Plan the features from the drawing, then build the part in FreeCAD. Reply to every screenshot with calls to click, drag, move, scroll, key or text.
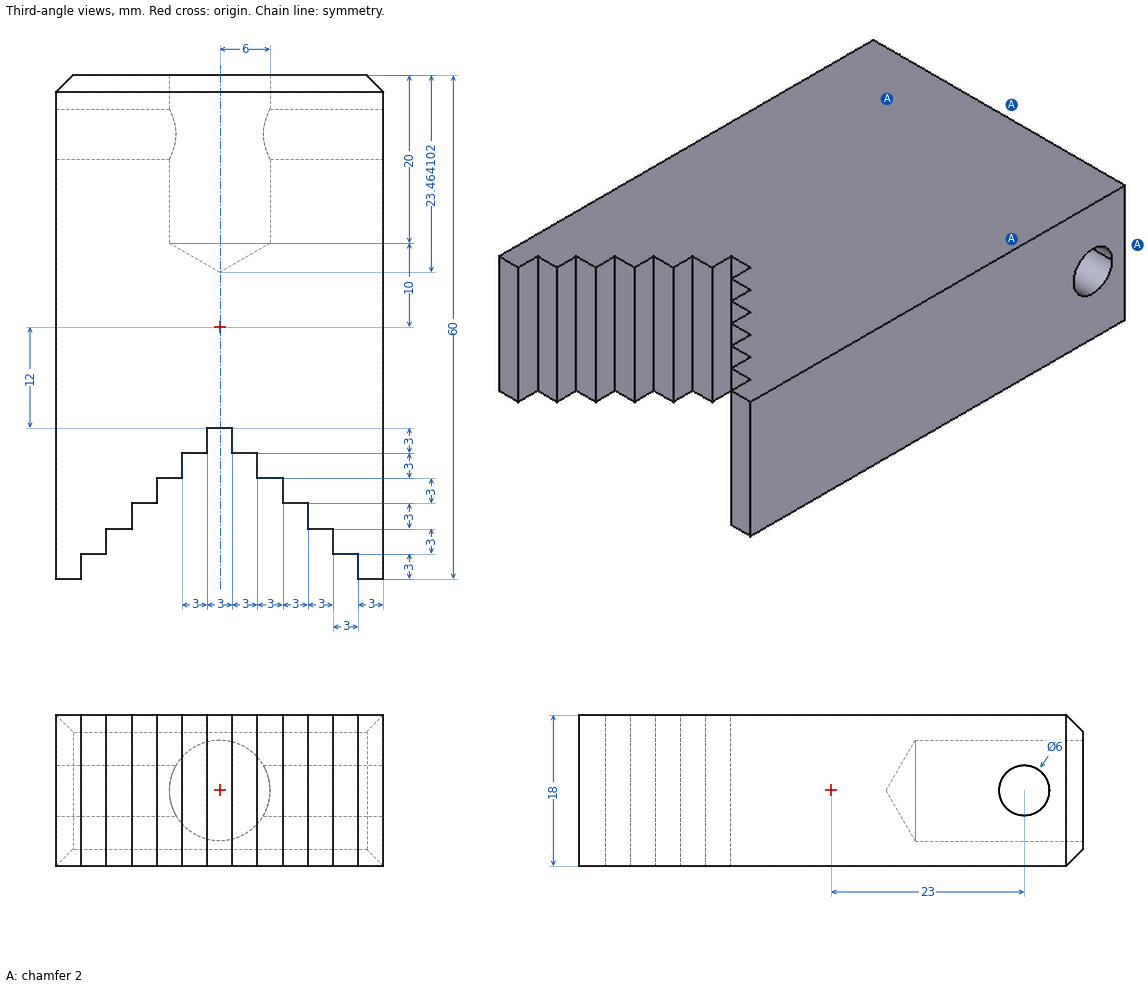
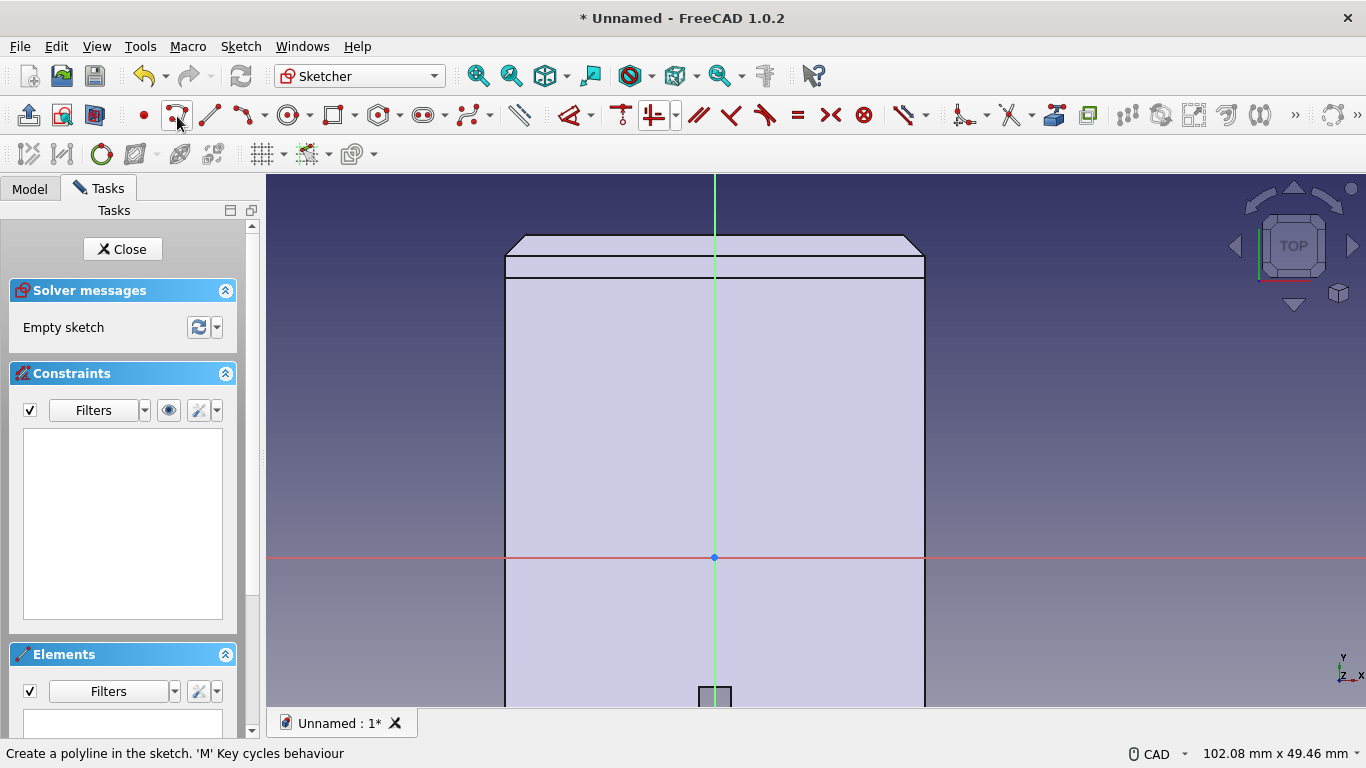
click(715, 487)
click(779, 450)
click(779, 235)
click(724, 235)
click(715, 488)
key(Escape)
key(Escape)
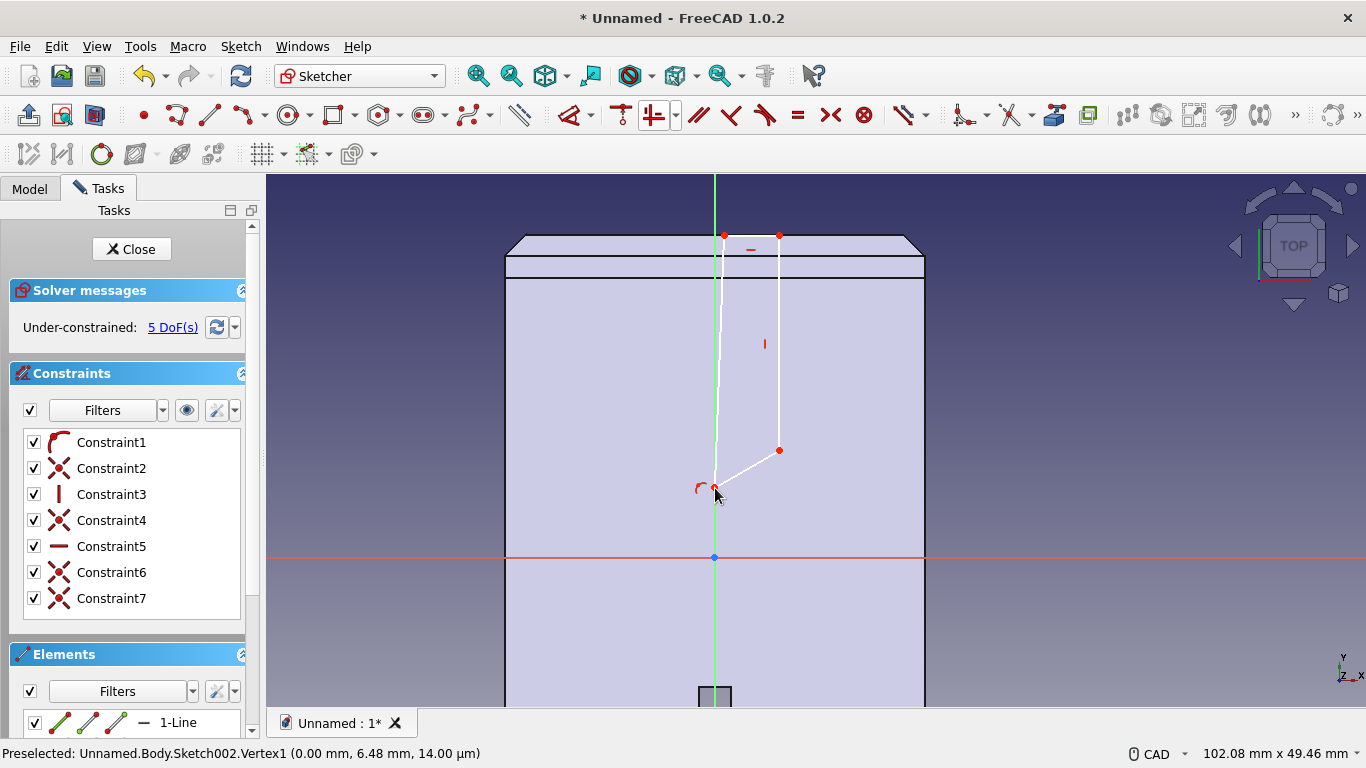
click(718, 412)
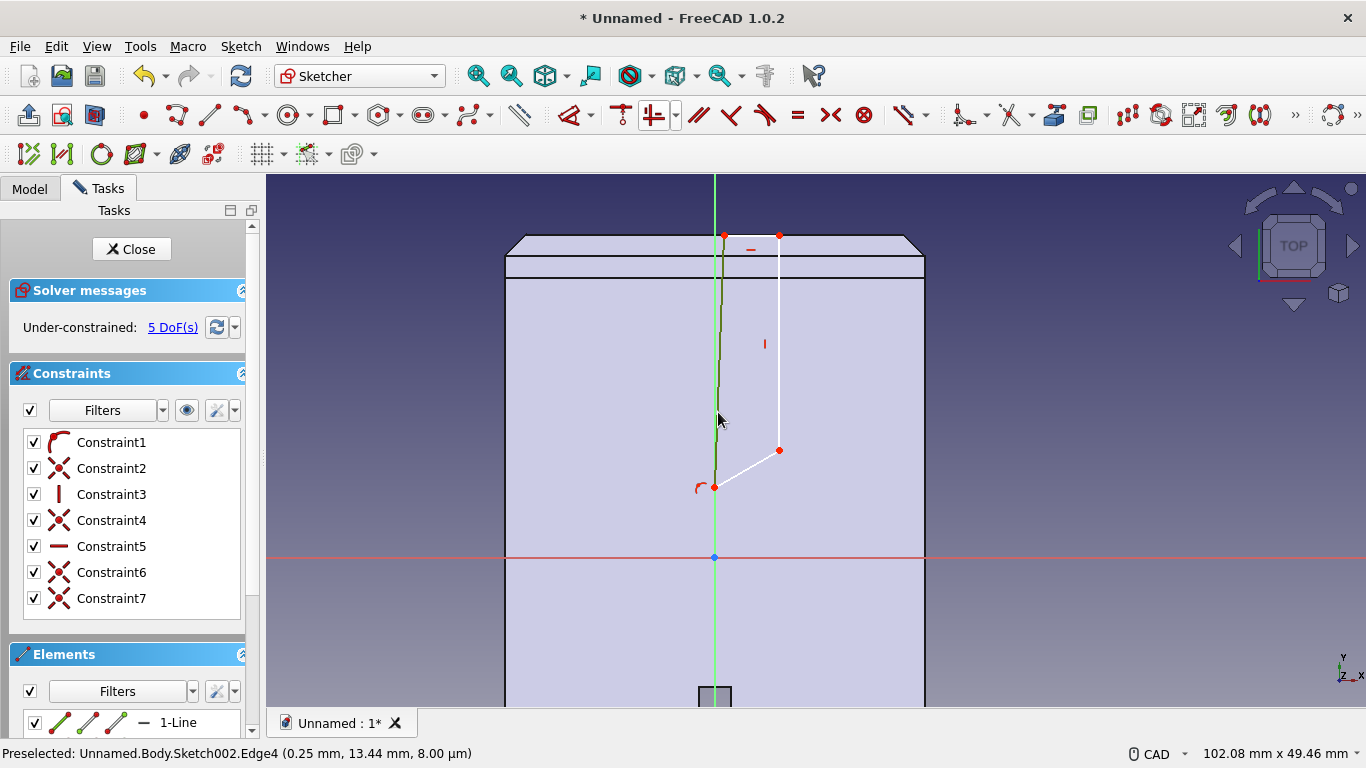
click(676, 116)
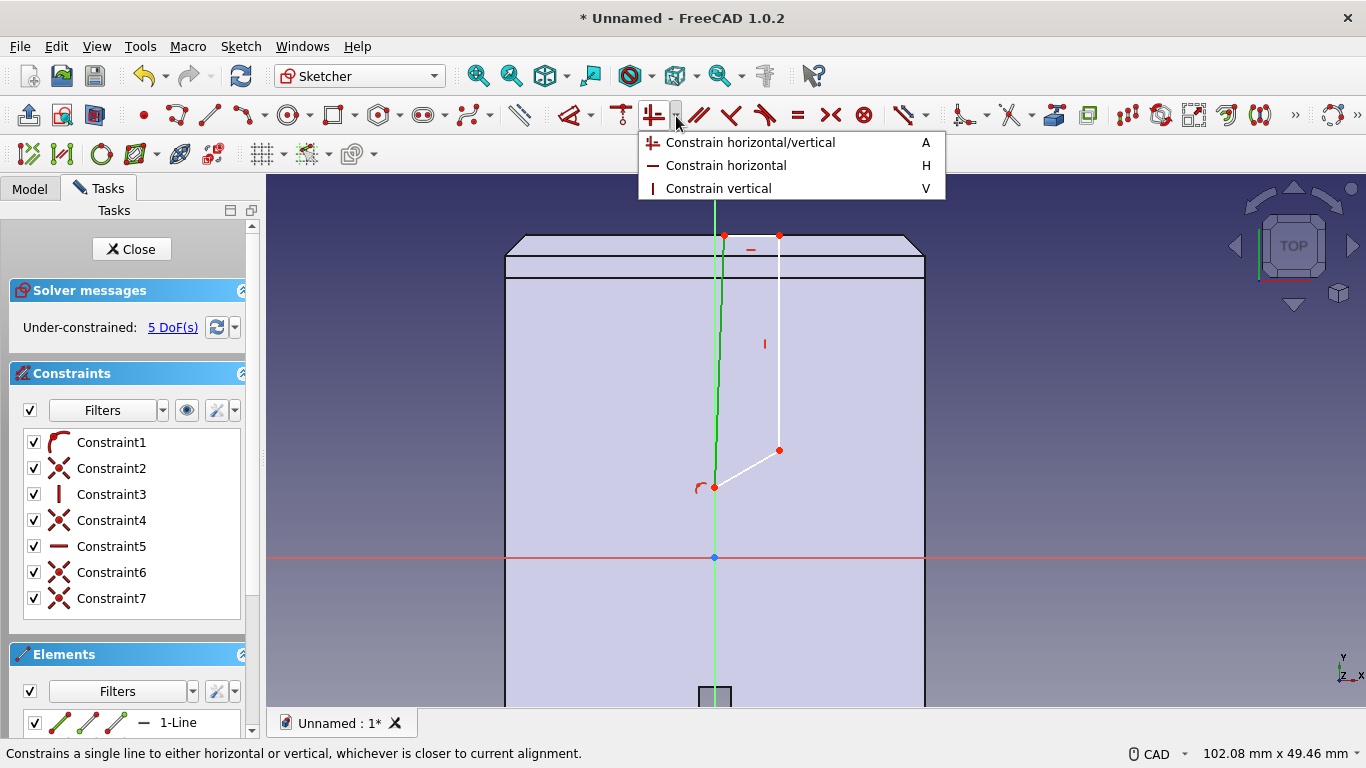
click(792, 188)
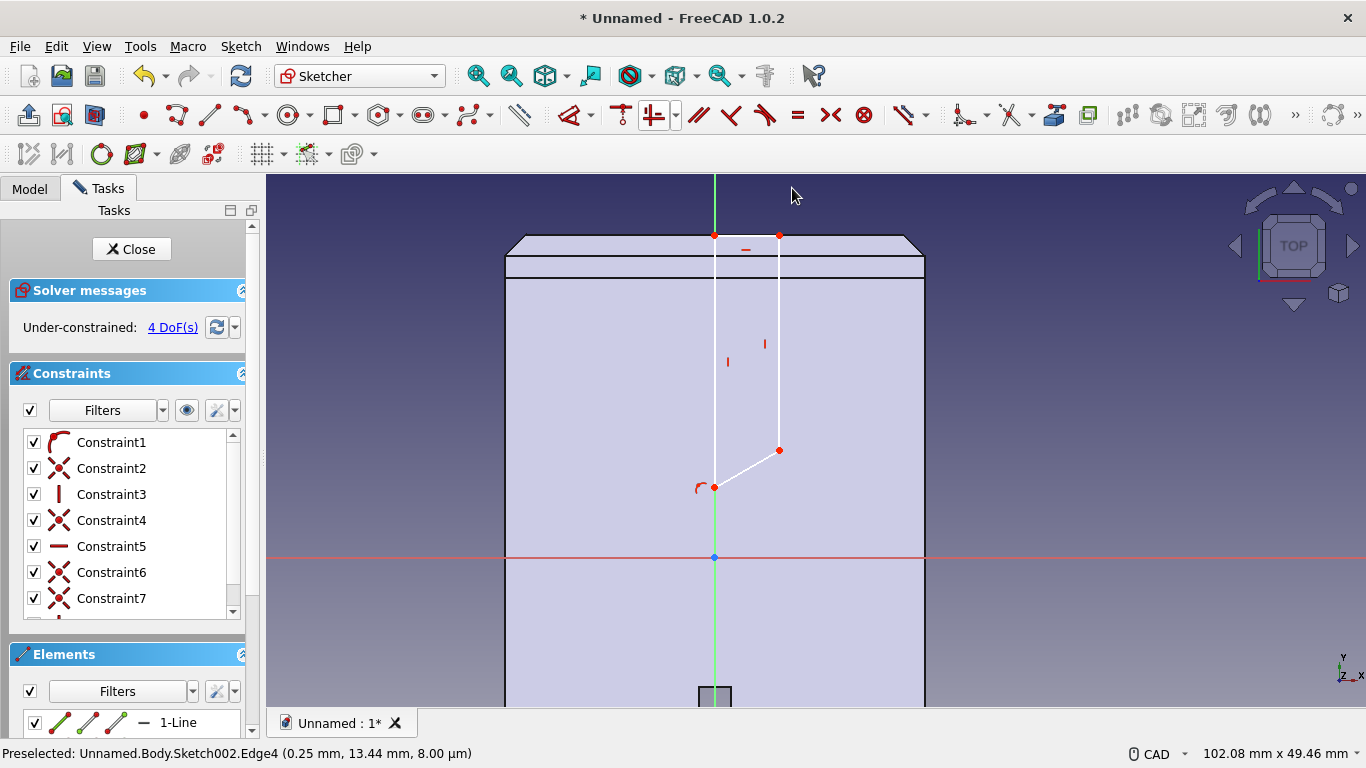
click(568, 116)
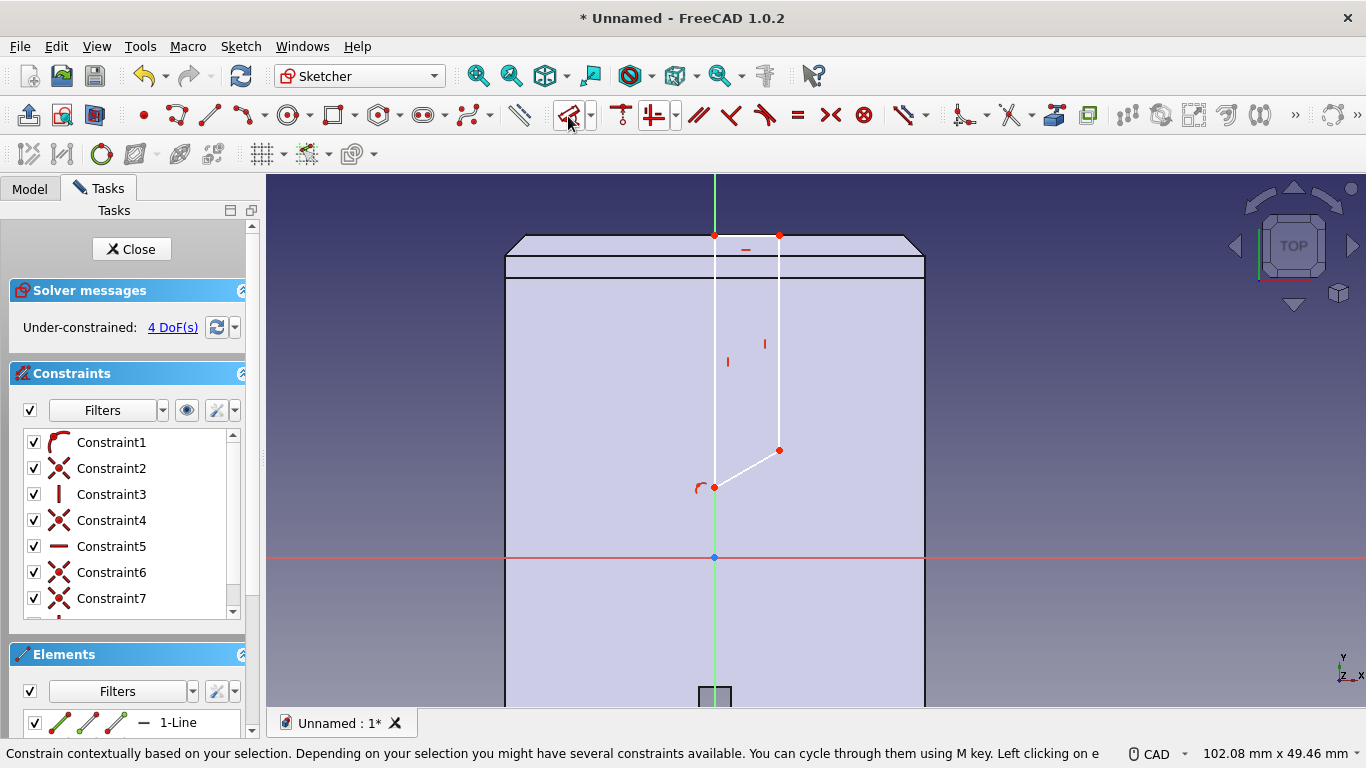
click(760, 236)
click(747, 270)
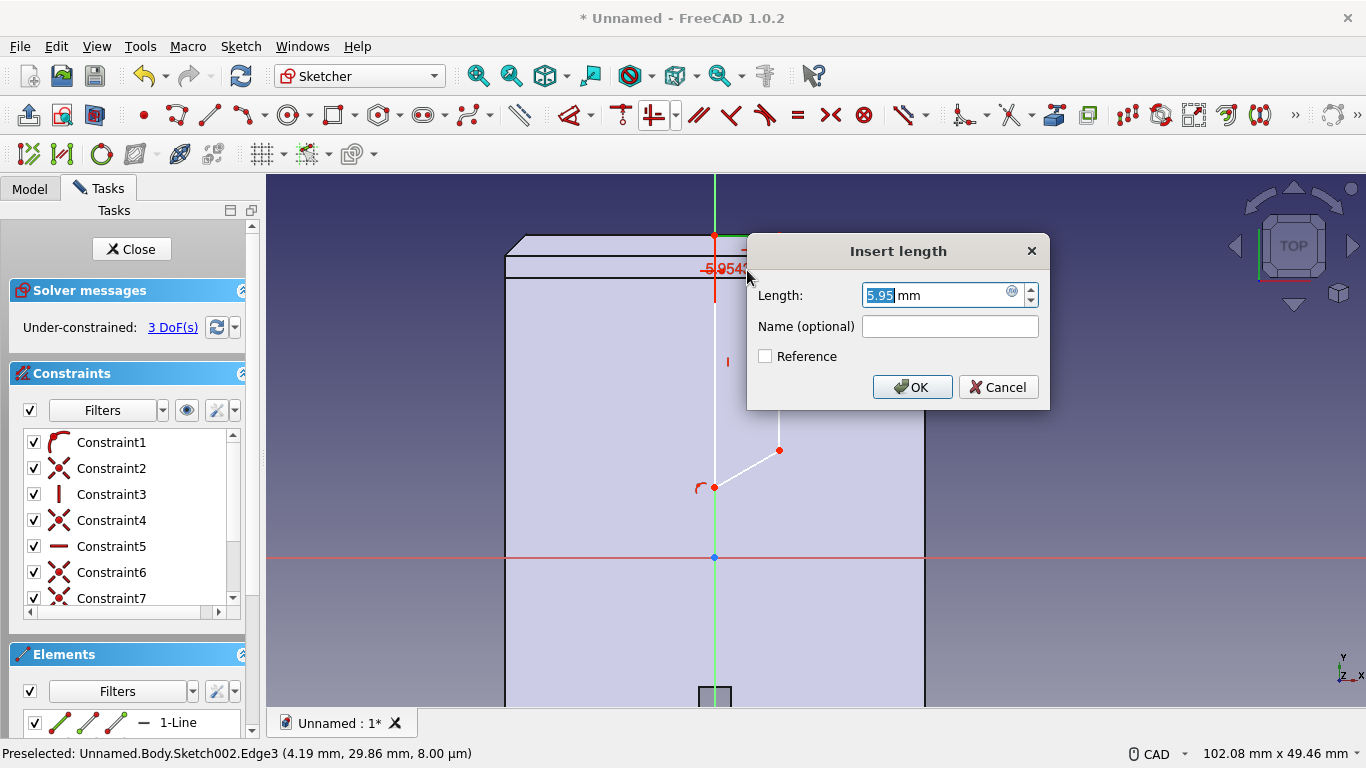
text(6)
key(Return)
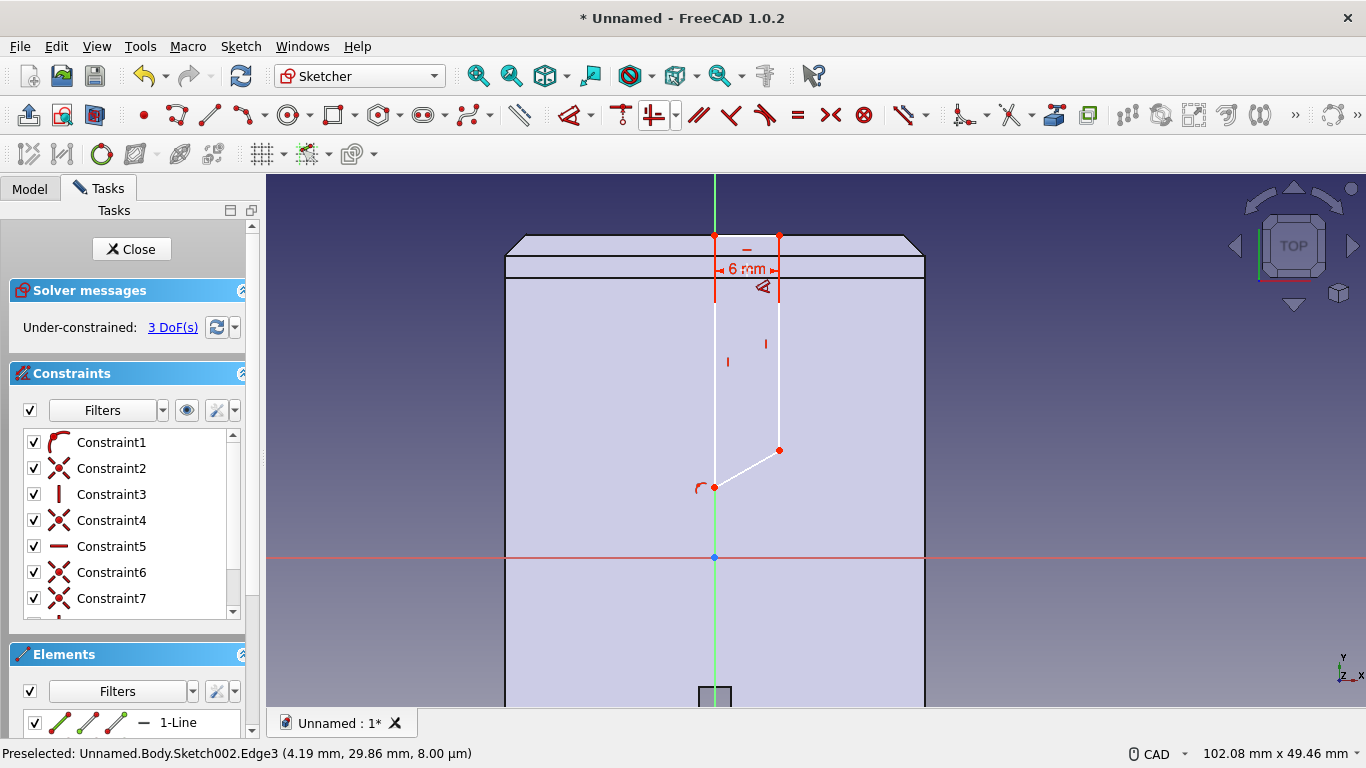
click(779, 386)
click(813, 343)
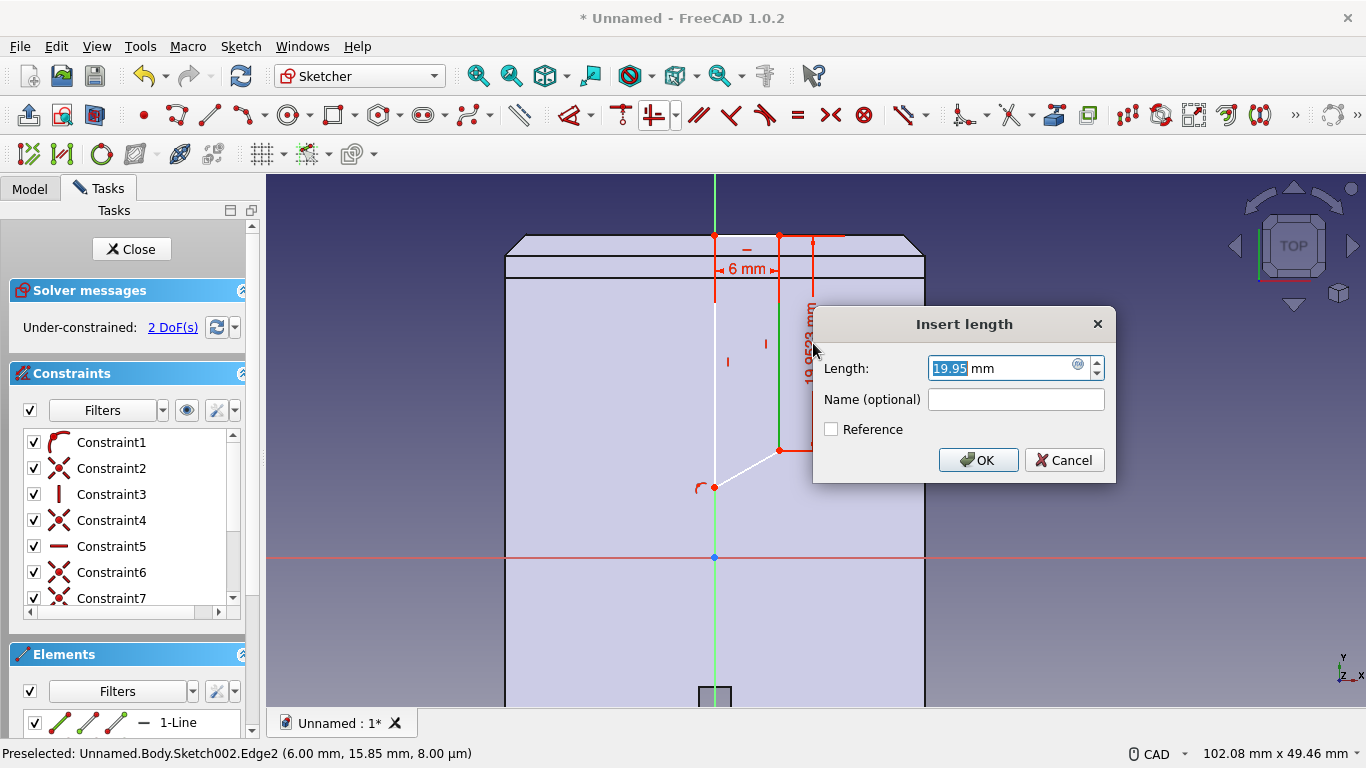
text(20)
key(Return)